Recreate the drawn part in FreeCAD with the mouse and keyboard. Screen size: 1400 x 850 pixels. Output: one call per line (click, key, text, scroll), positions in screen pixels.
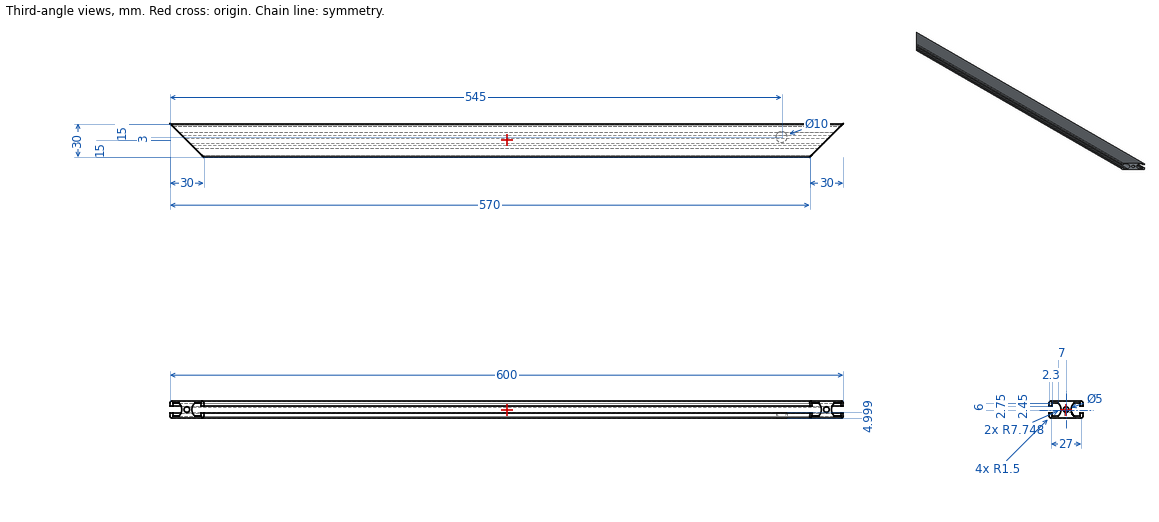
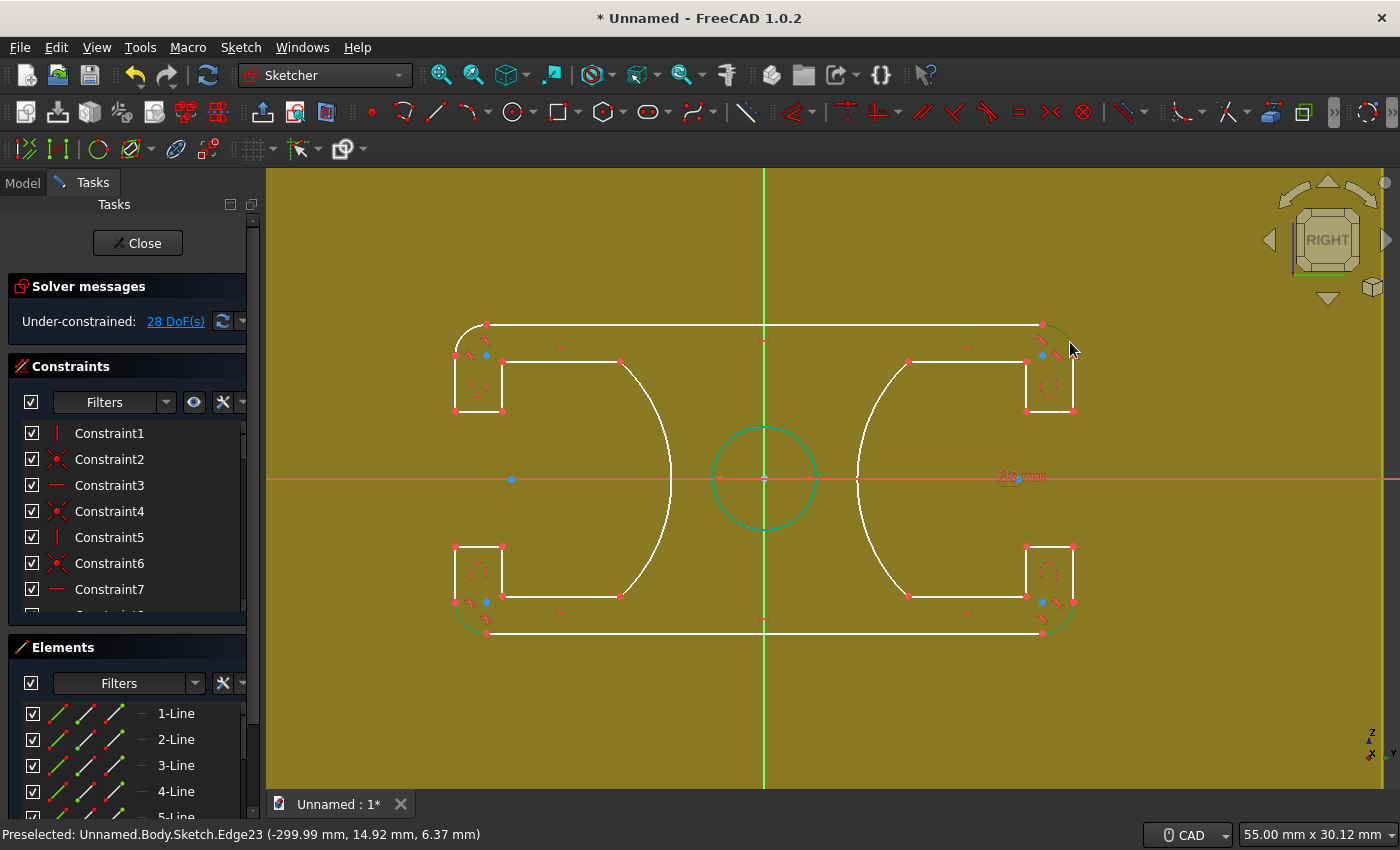
click(472, 328)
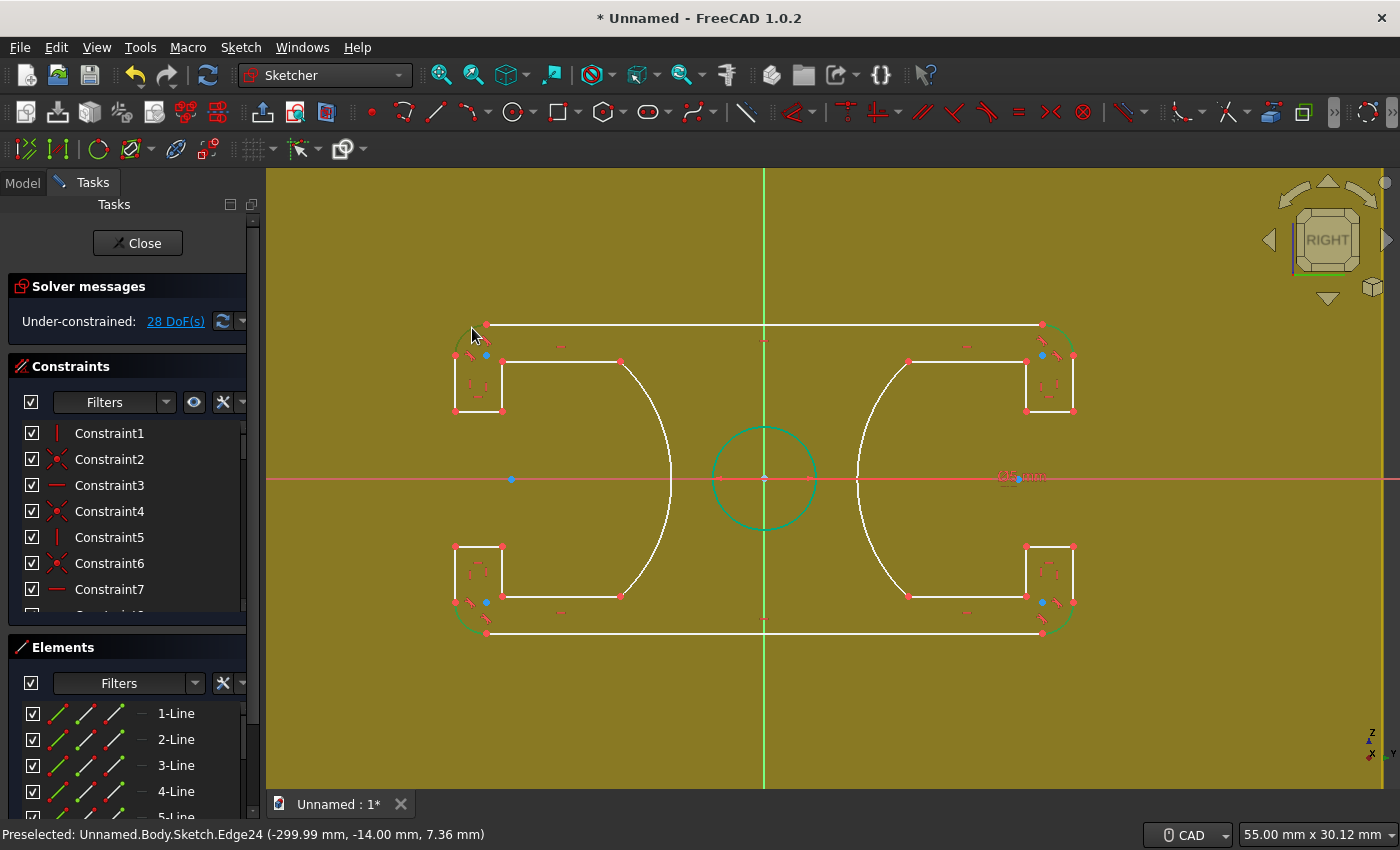
key(e)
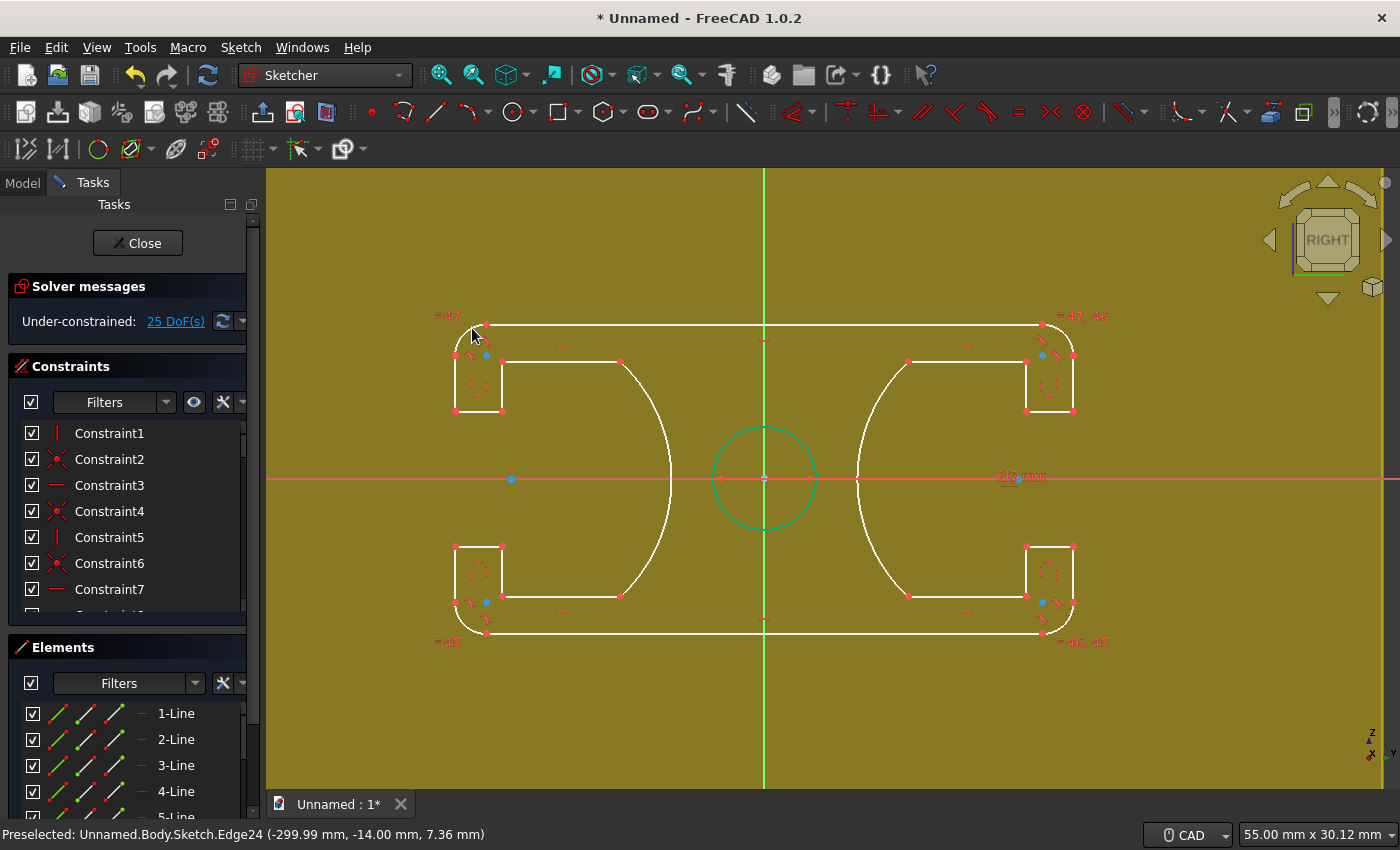
click(663, 531)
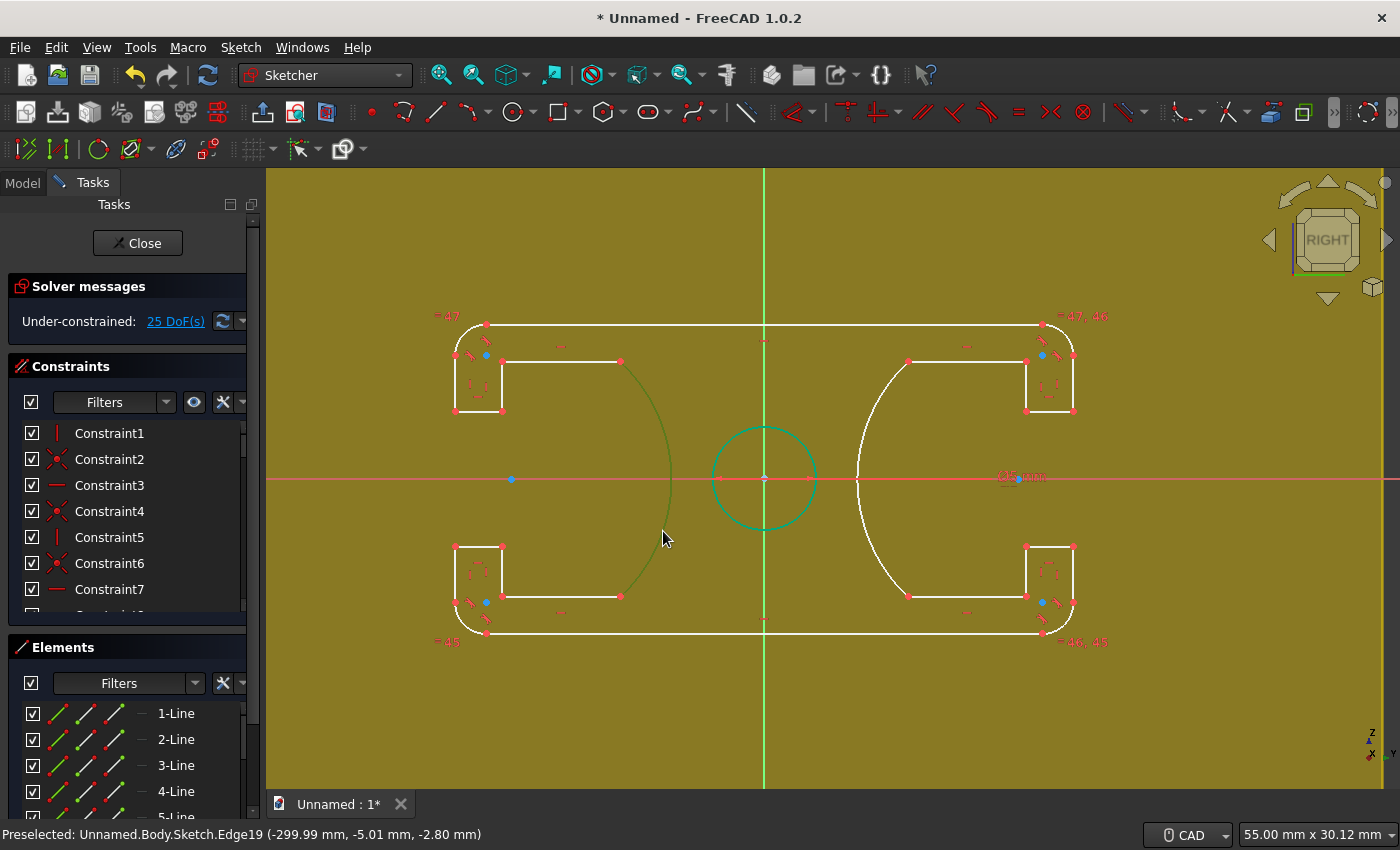
click(866, 428)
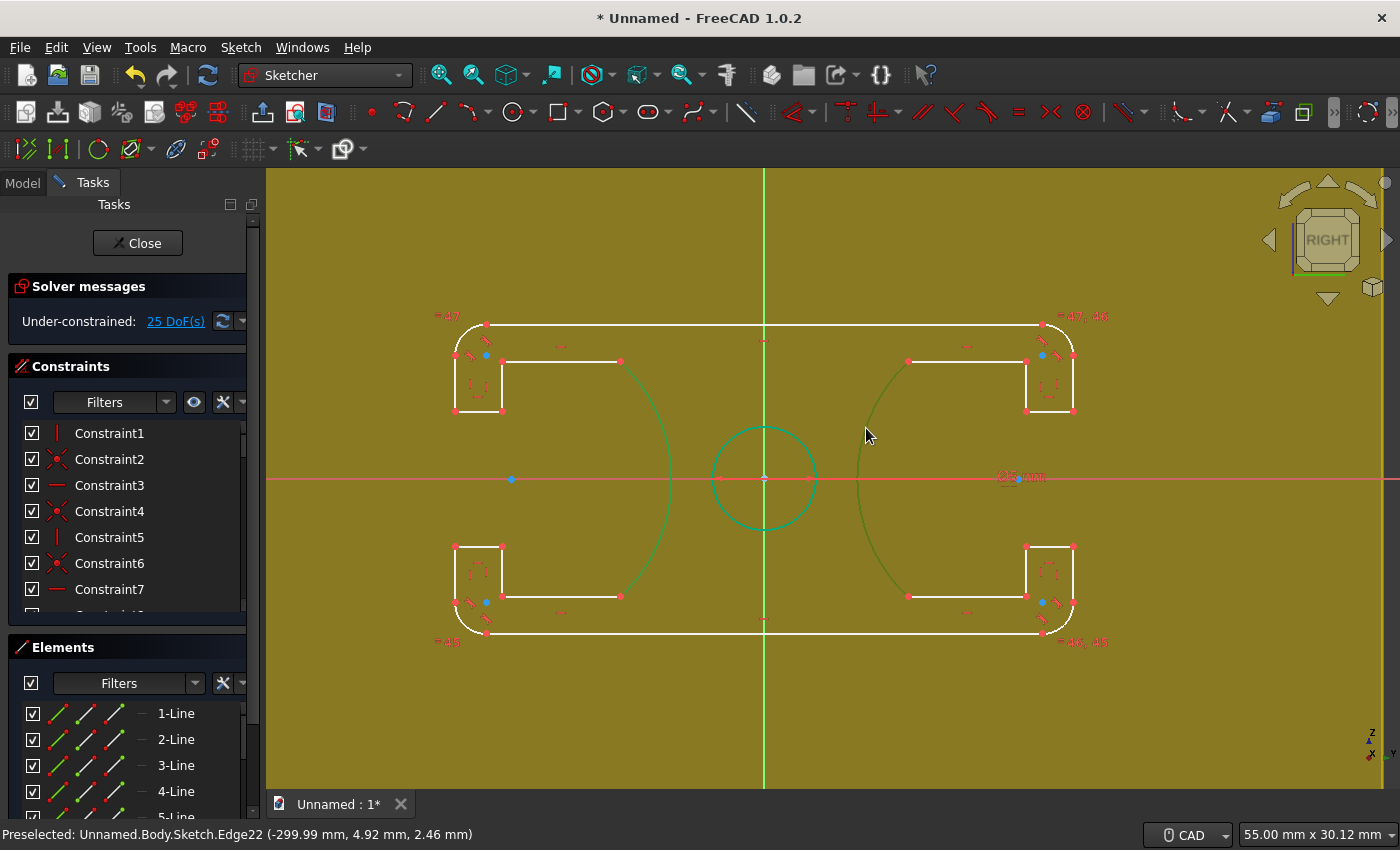
key(e)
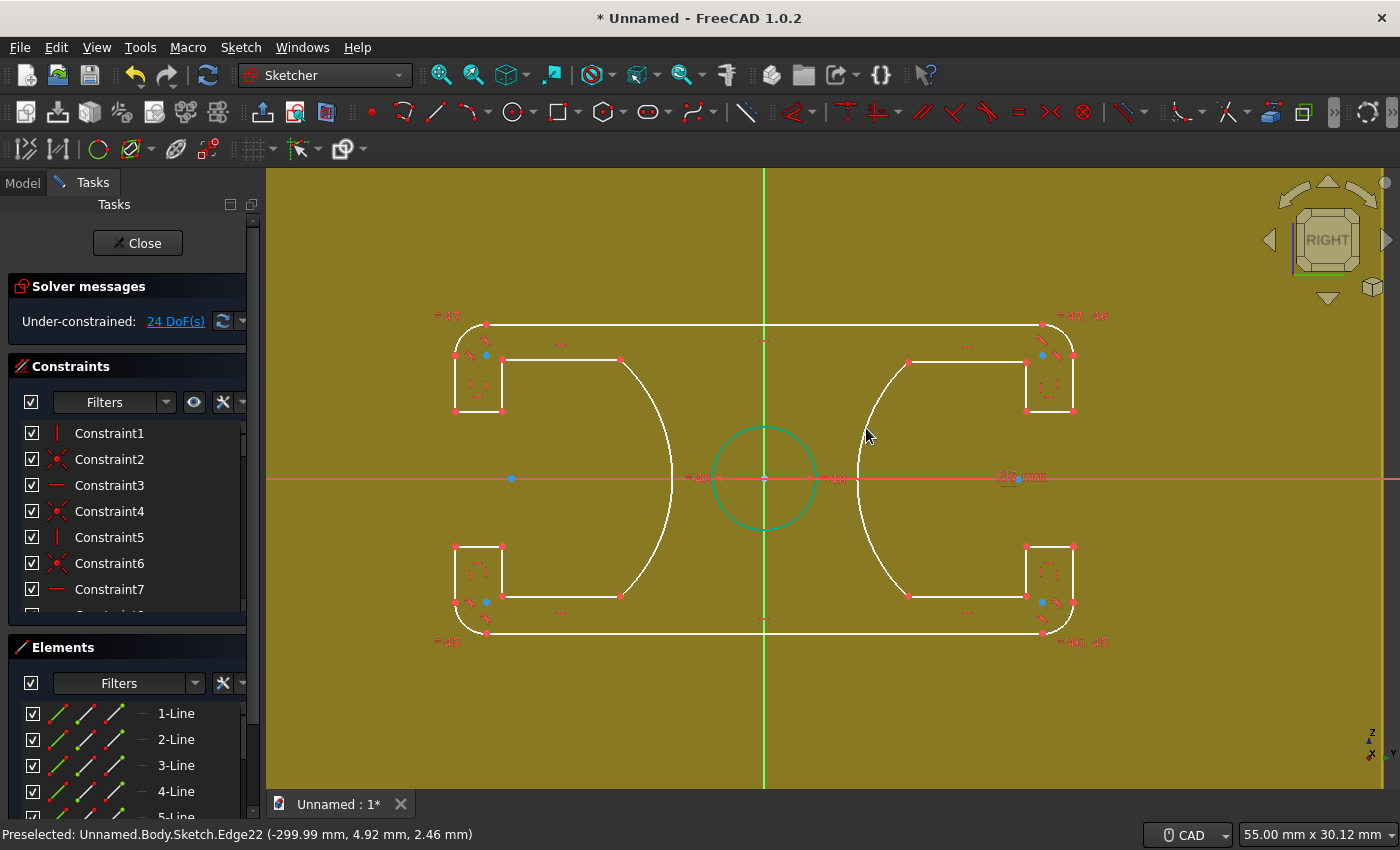
click(511, 478)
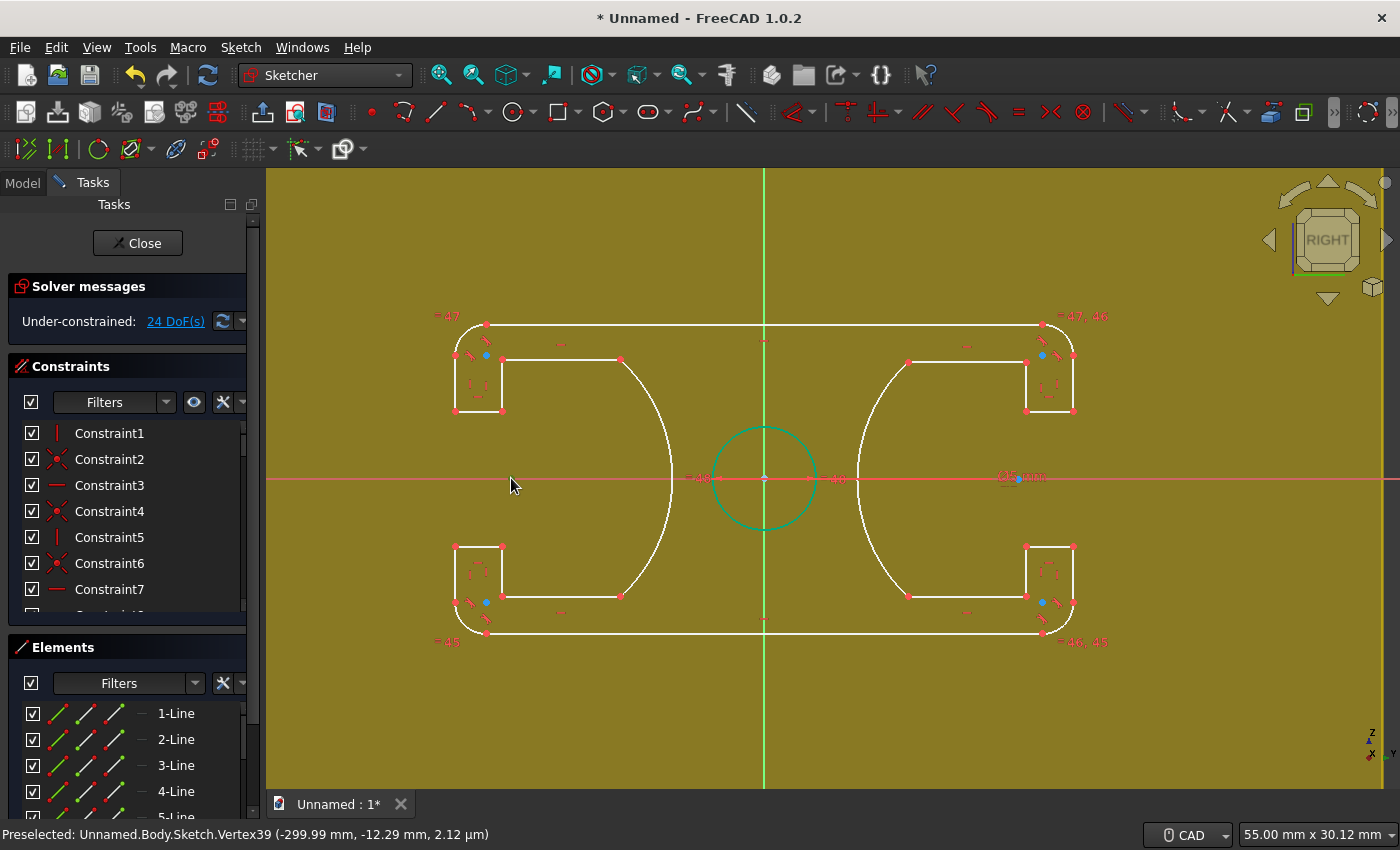
click(361, 478)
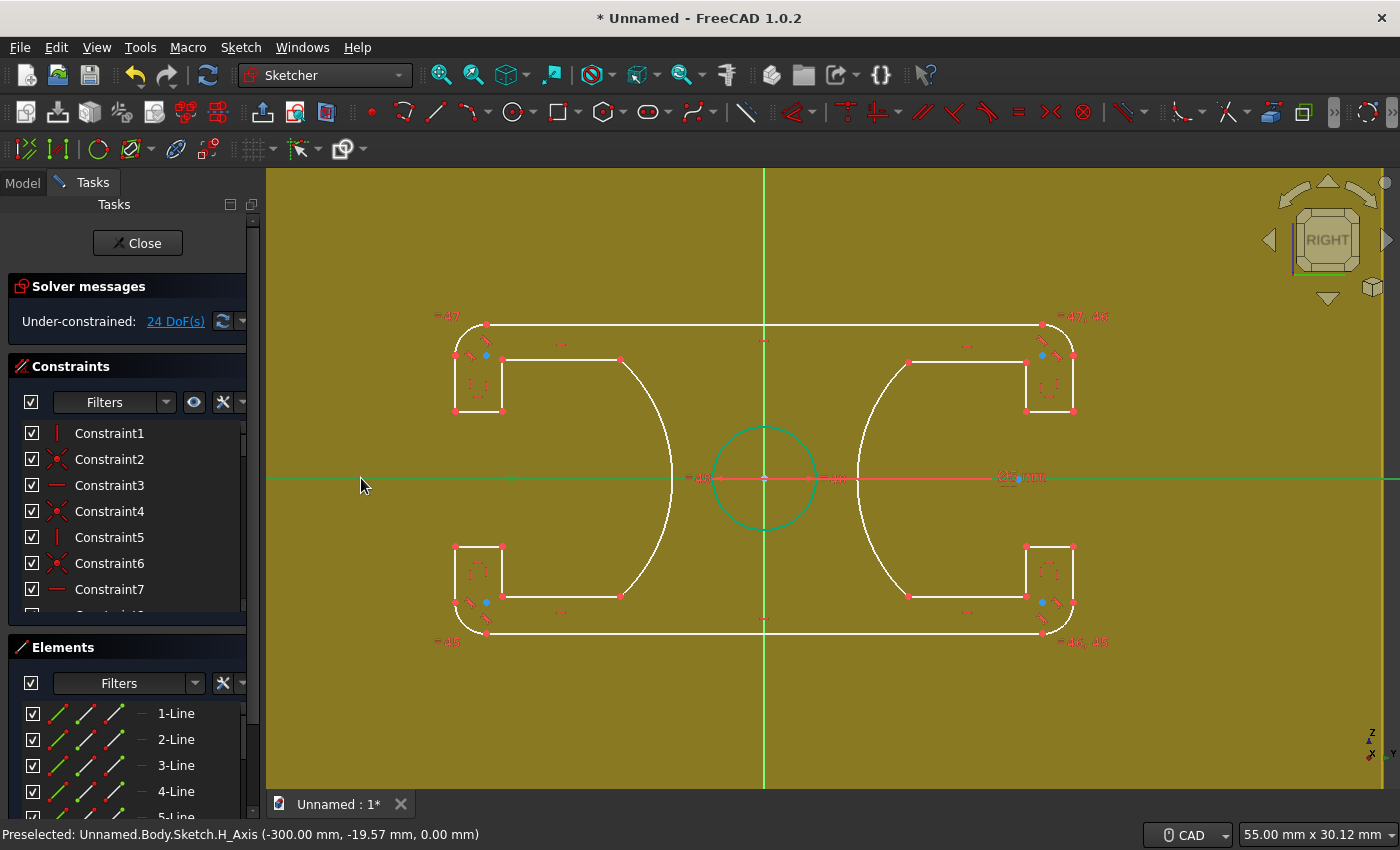
click(846, 112)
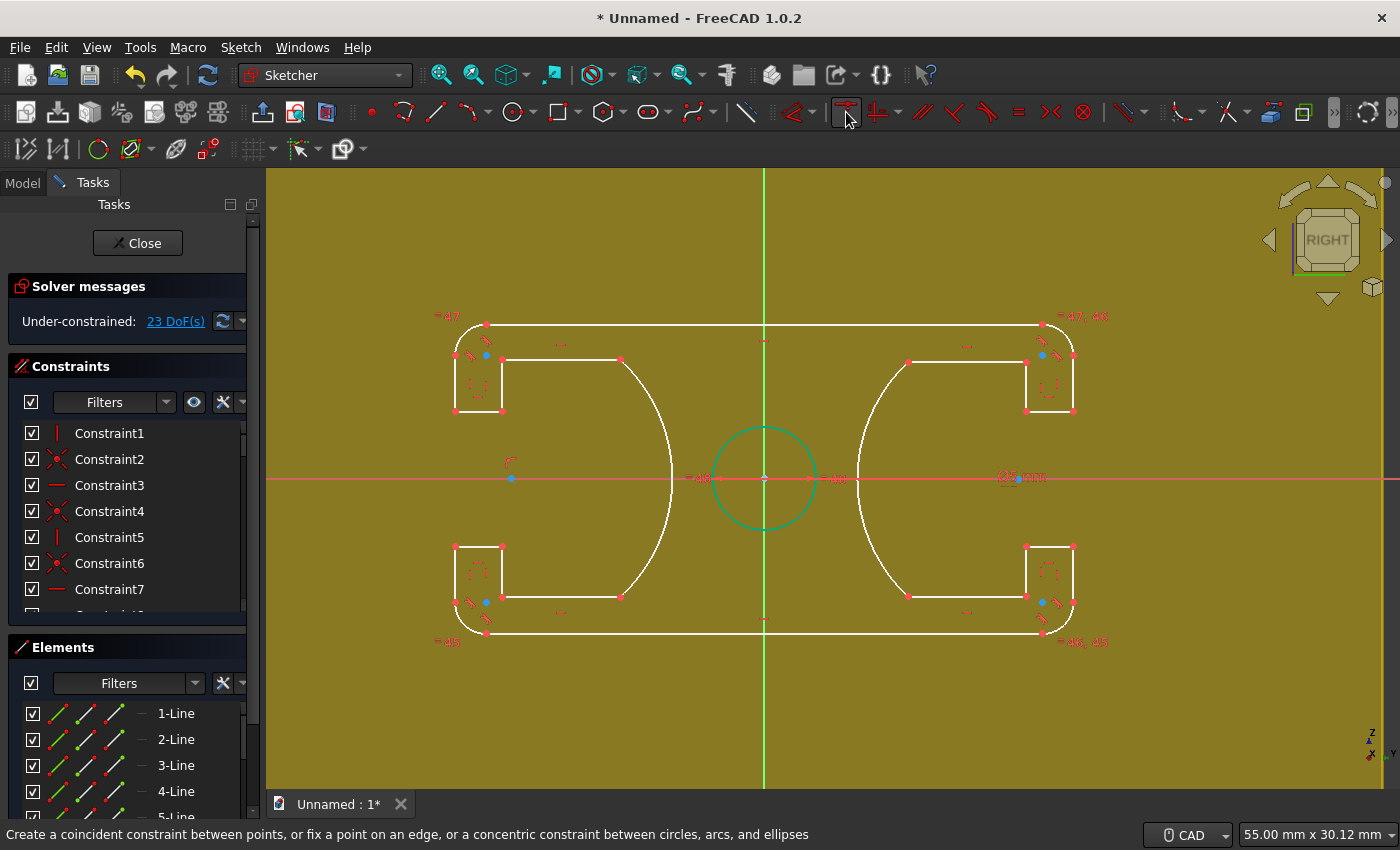
click(1019, 480)